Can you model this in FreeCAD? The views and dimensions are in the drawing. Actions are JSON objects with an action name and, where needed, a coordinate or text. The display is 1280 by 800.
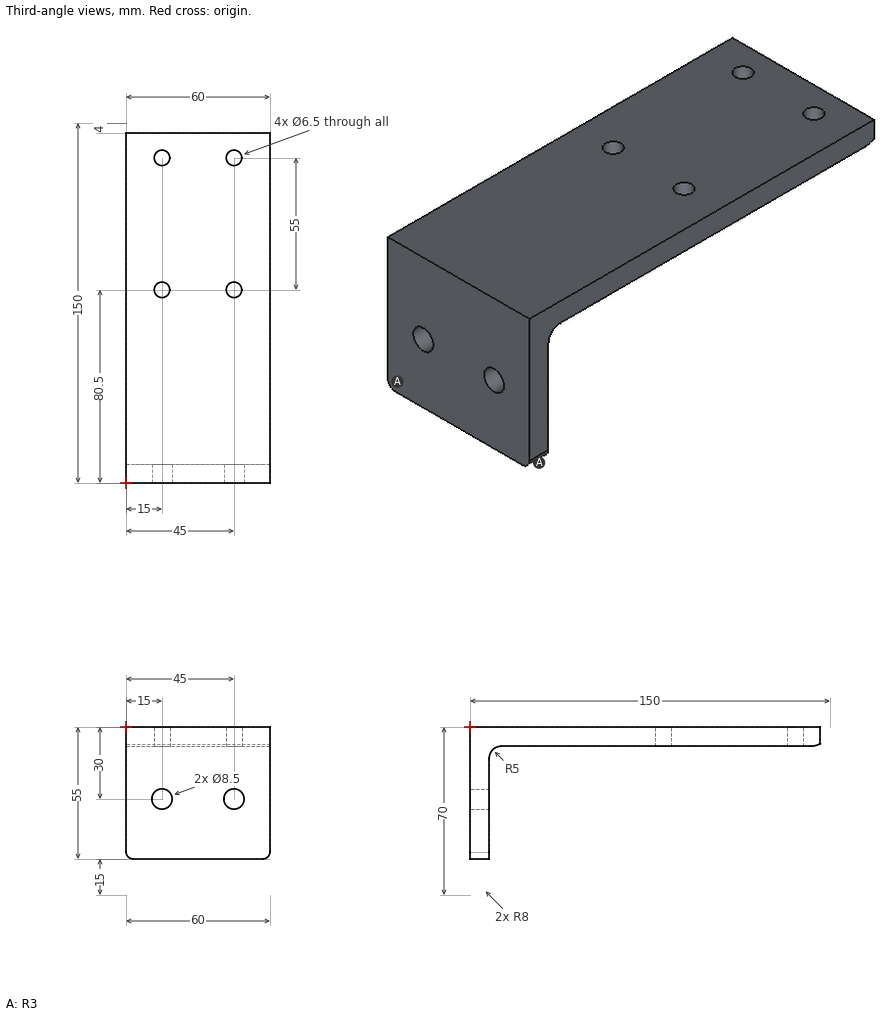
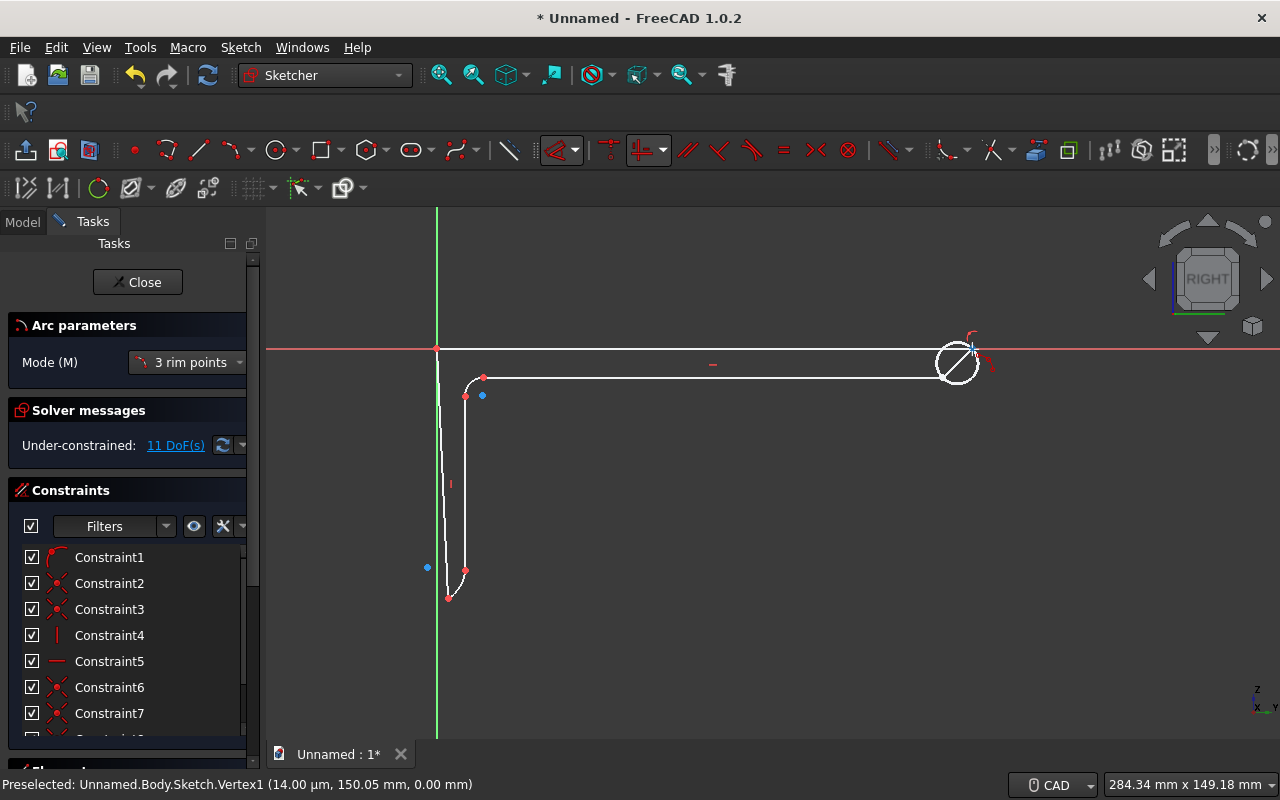
{"action": "scroll", "coordinate": [964, 369], "scroll_direction": "up", "scroll_amount": 4}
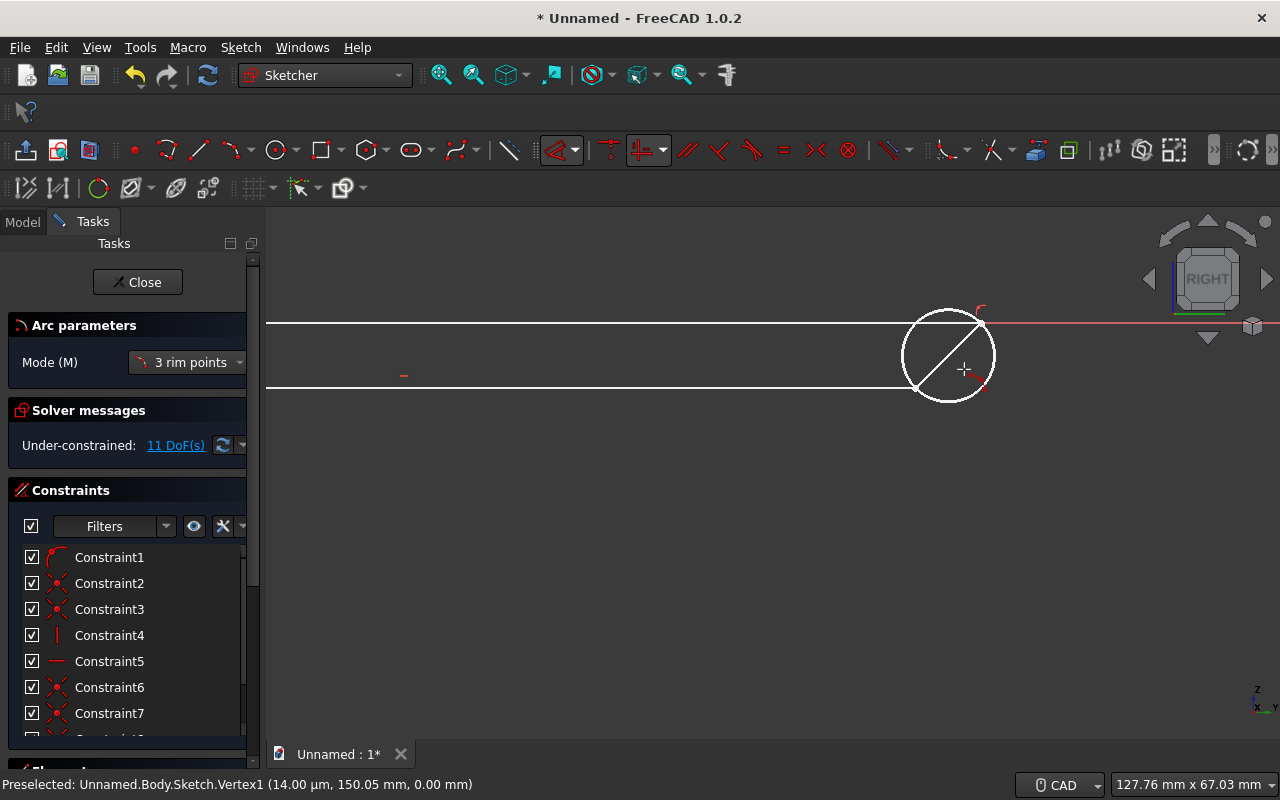
{"action": "left_click", "coordinate": [962, 368]}
{"action": "key", "text": "Escape"}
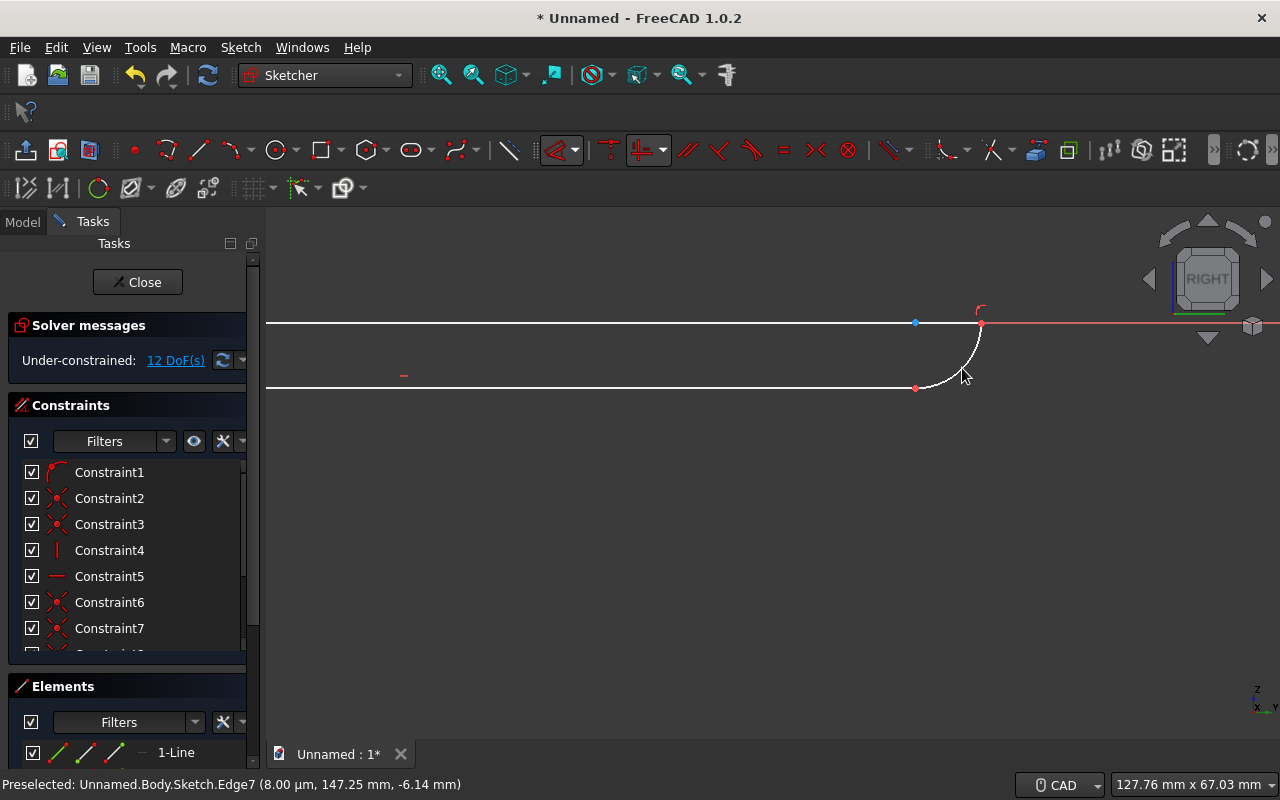
{"action": "scroll", "coordinate": [965, 369], "scroll_direction": "down", "scroll_amount": 4}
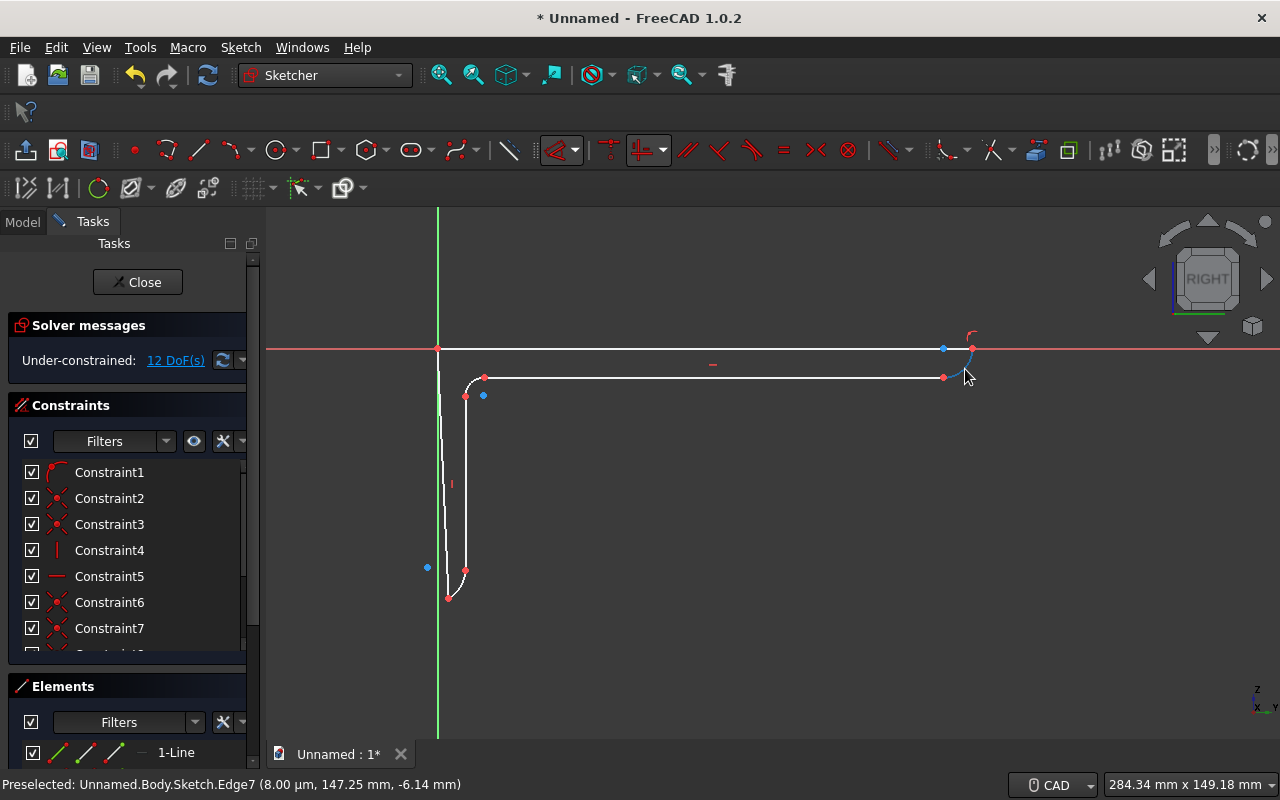
{"action": "left_click", "coordinate": [466, 518]}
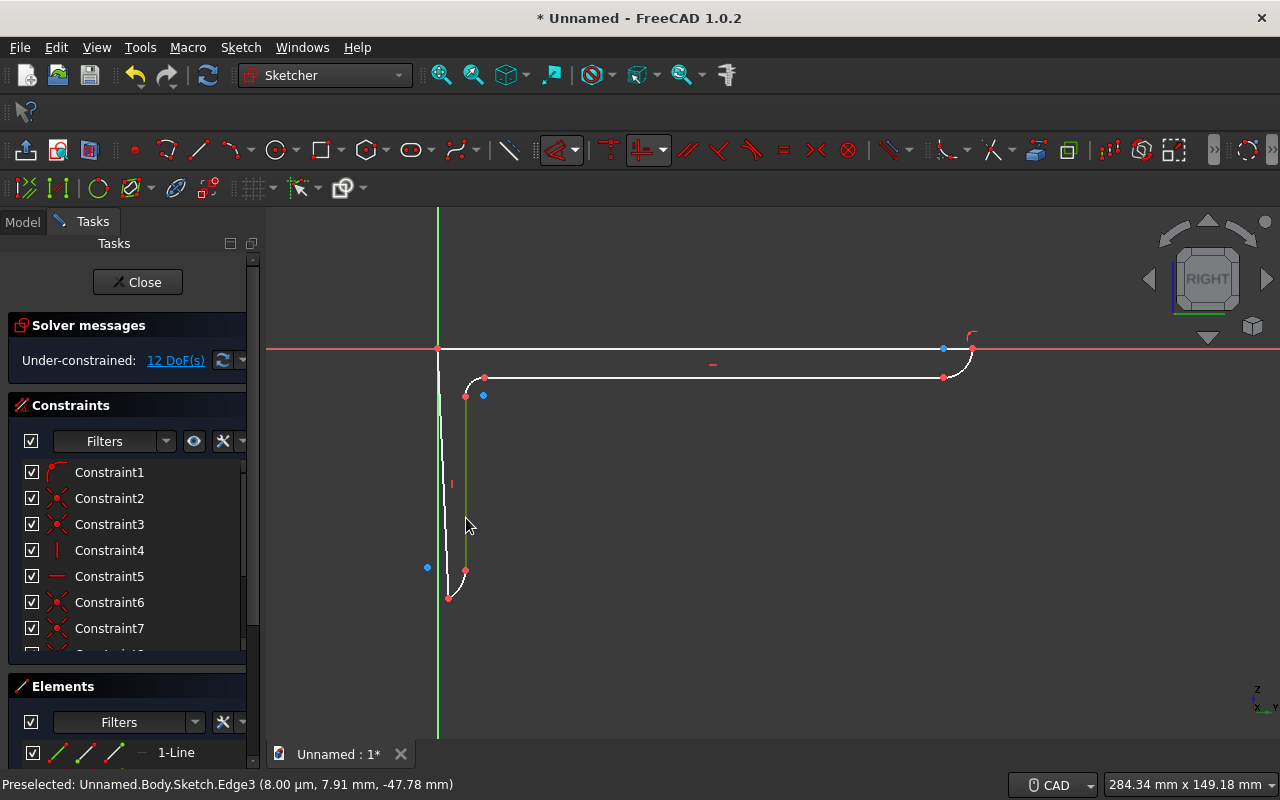
{"action": "scroll", "coordinate": [463, 581], "scroll_direction": "up", "scroll_amount": 2}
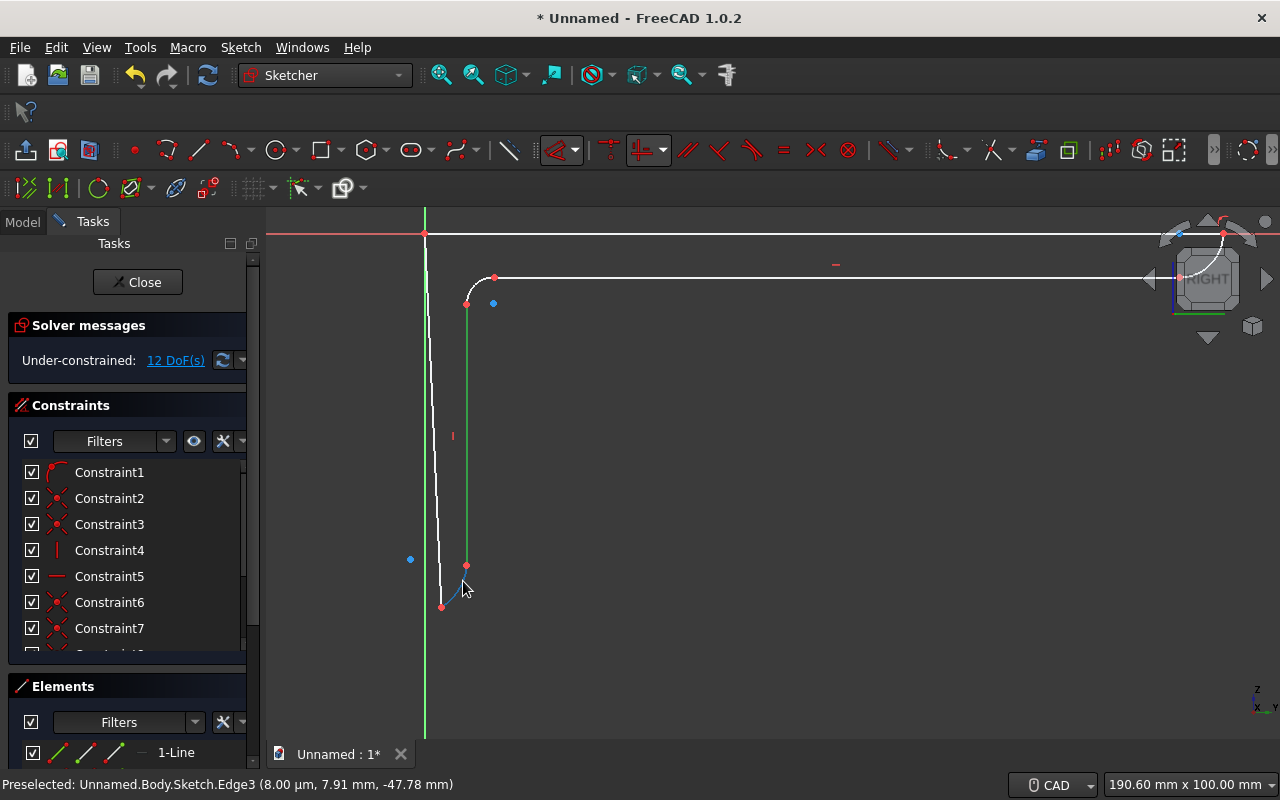
{"action": "left_click", "coordinate": [463, 580]}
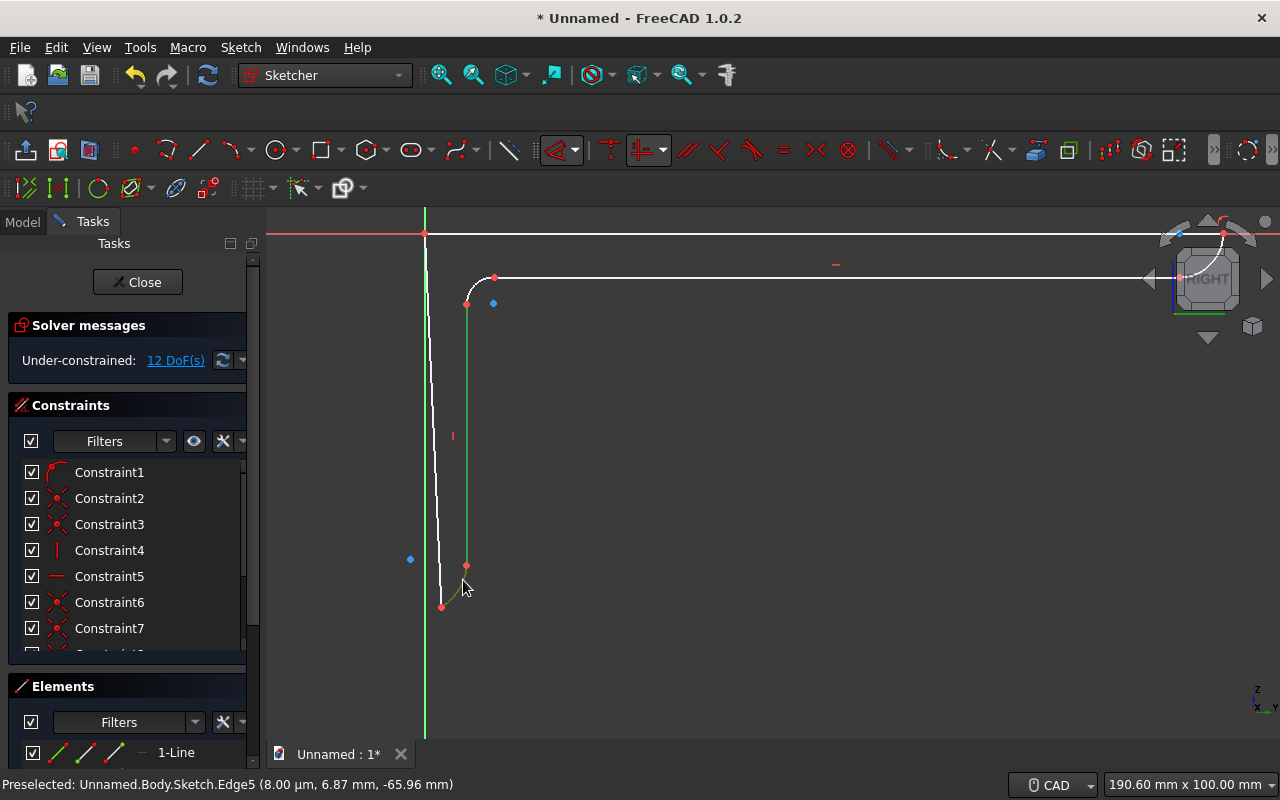
{"action": "key", "text": "t"}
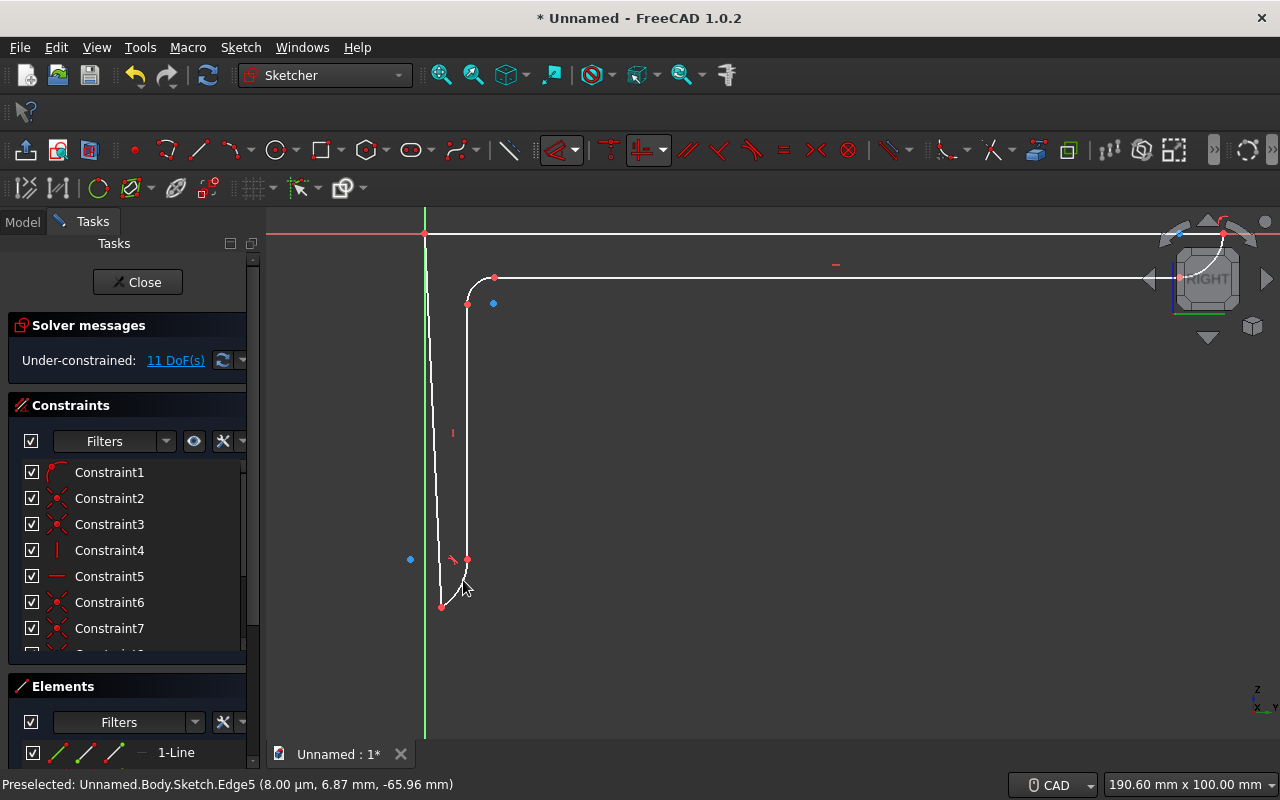
{"action": "left_click", "coordinate": [467, 483]}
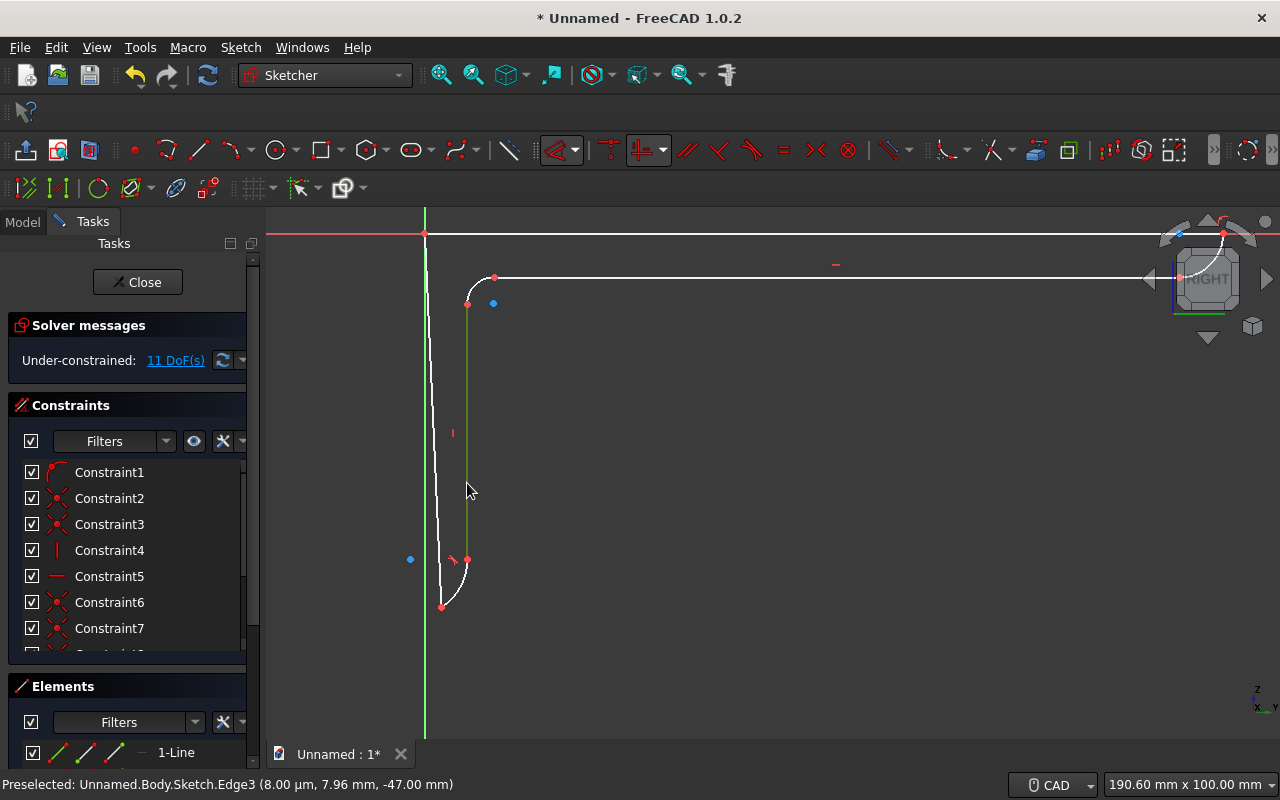
{"action": "left_click", "coordinate": [482, 280]}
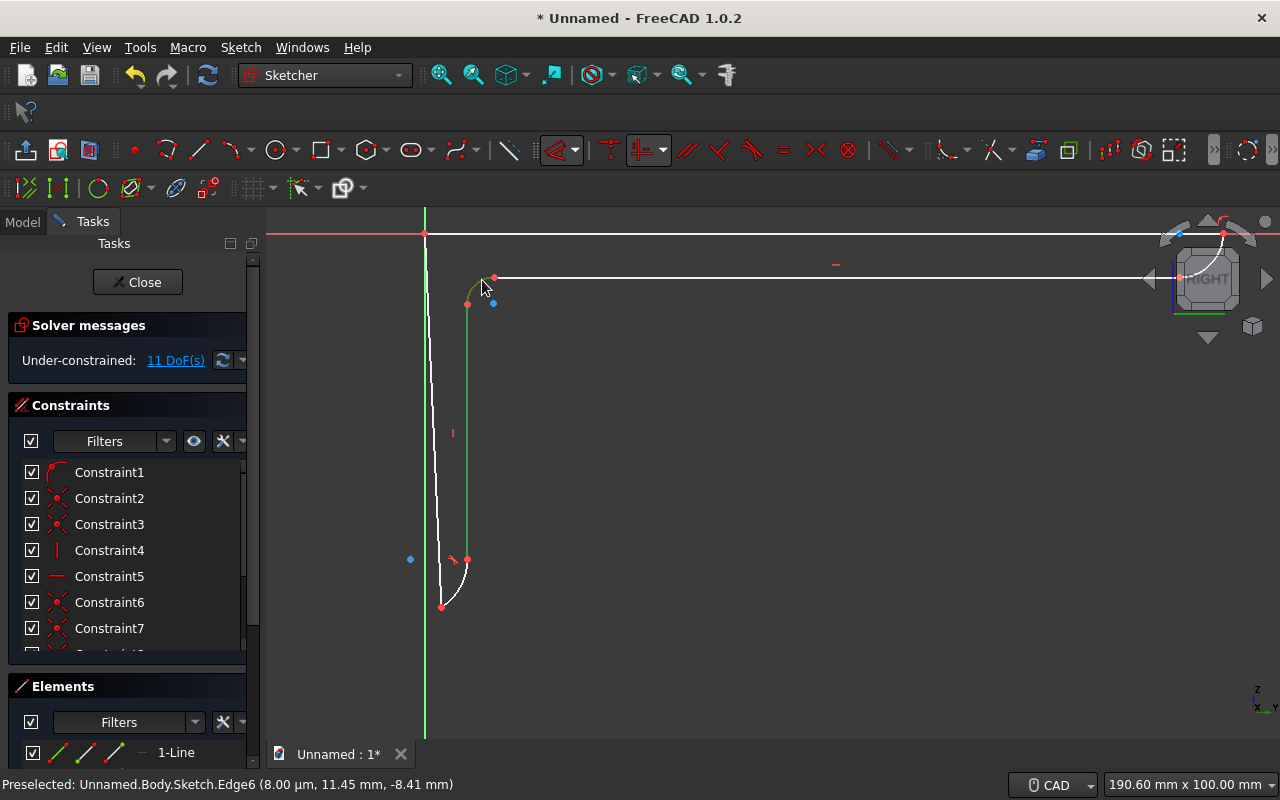
{"action": "key", "text": "t"}